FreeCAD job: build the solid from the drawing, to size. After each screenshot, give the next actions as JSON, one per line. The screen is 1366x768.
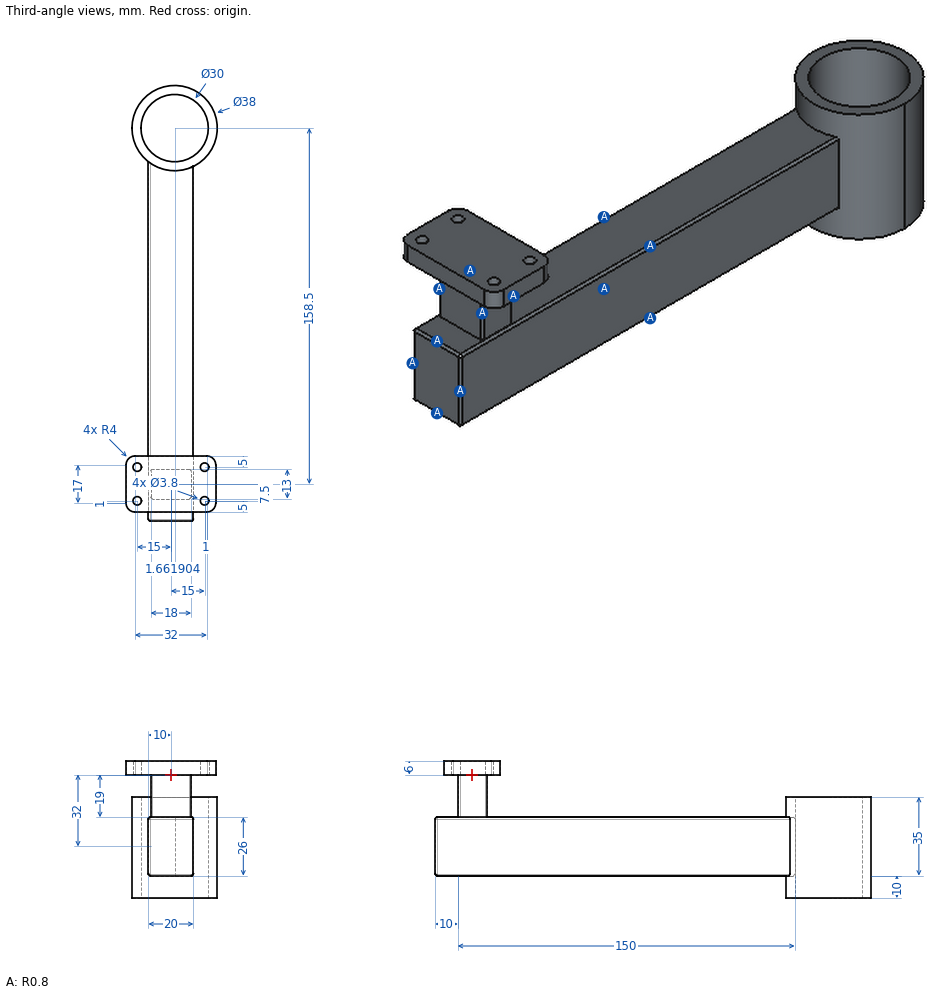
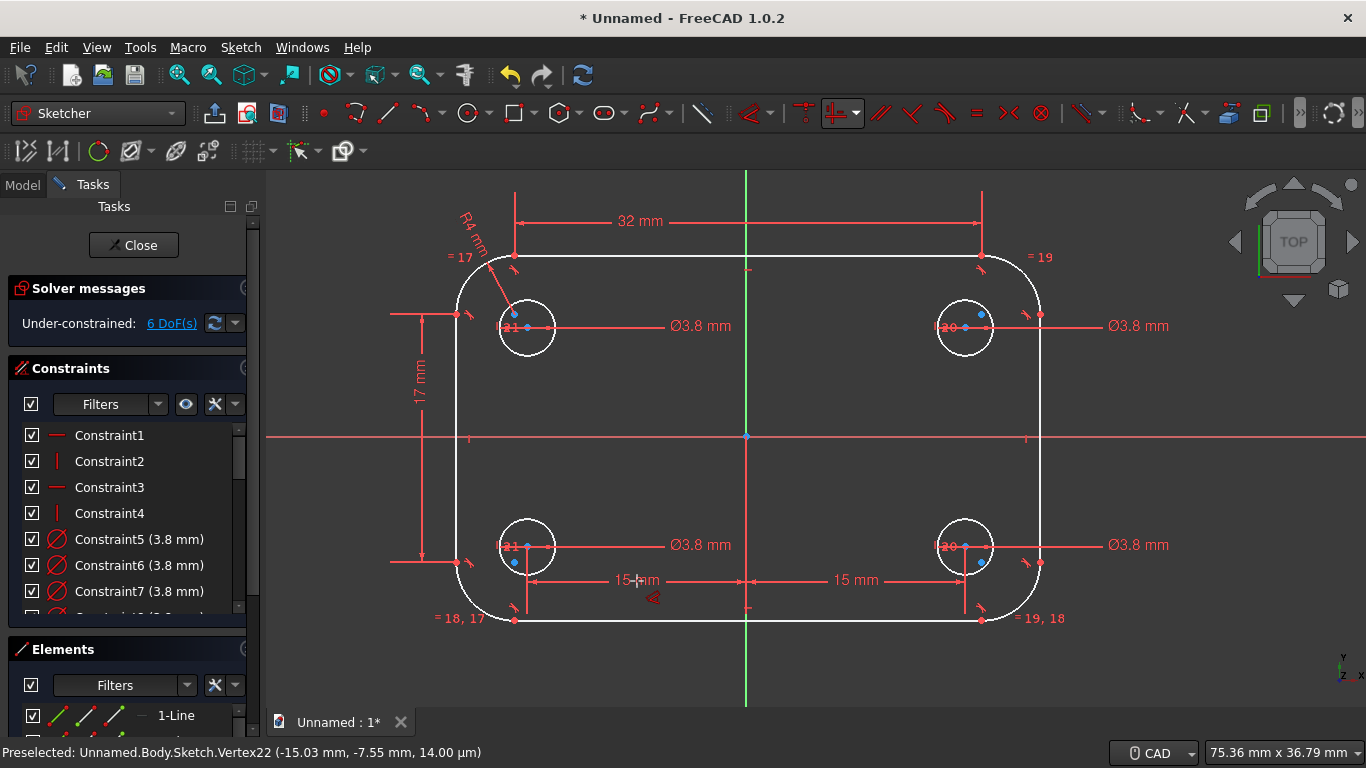
{"action": "scroll", "coordinate": [982, 621], "scroll_direction": "up", "scroll_amount": 6}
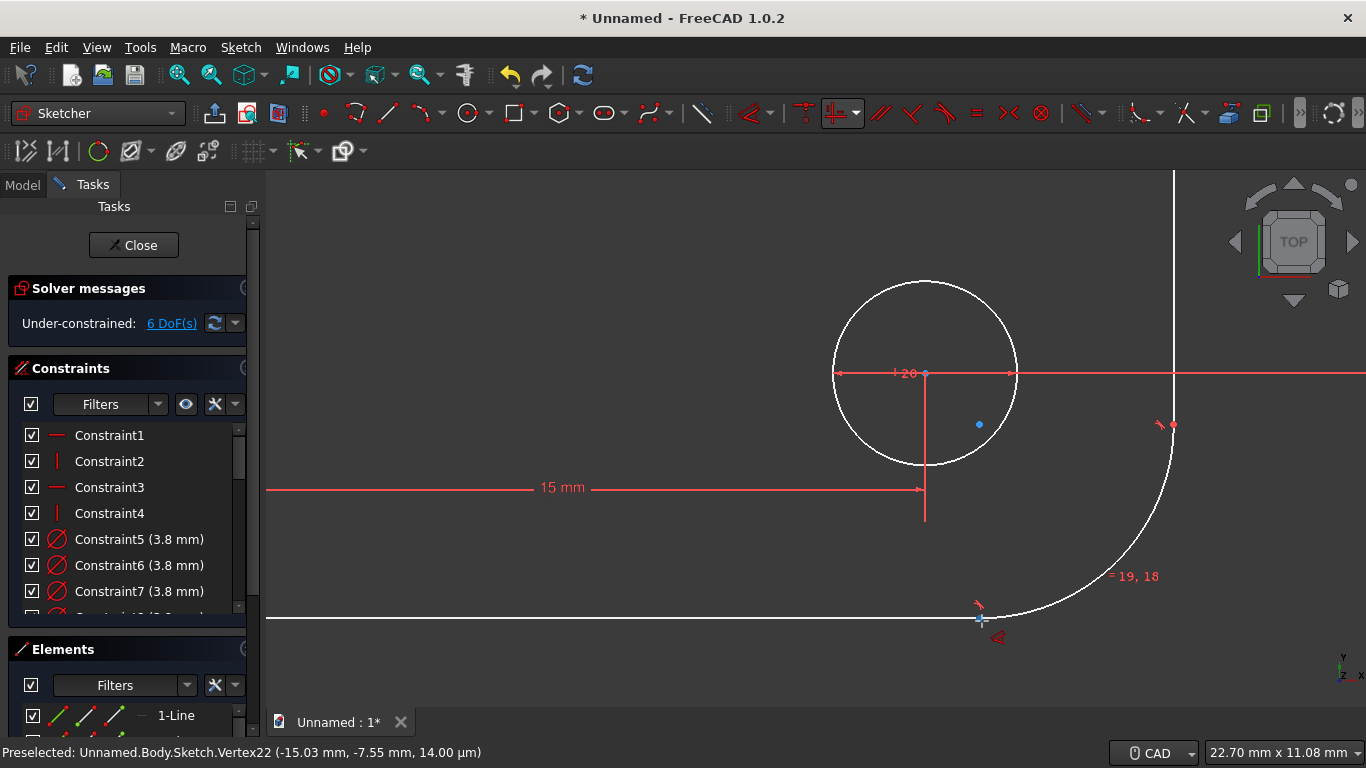
{"action": "left_click", "coordinate": [980, 618]}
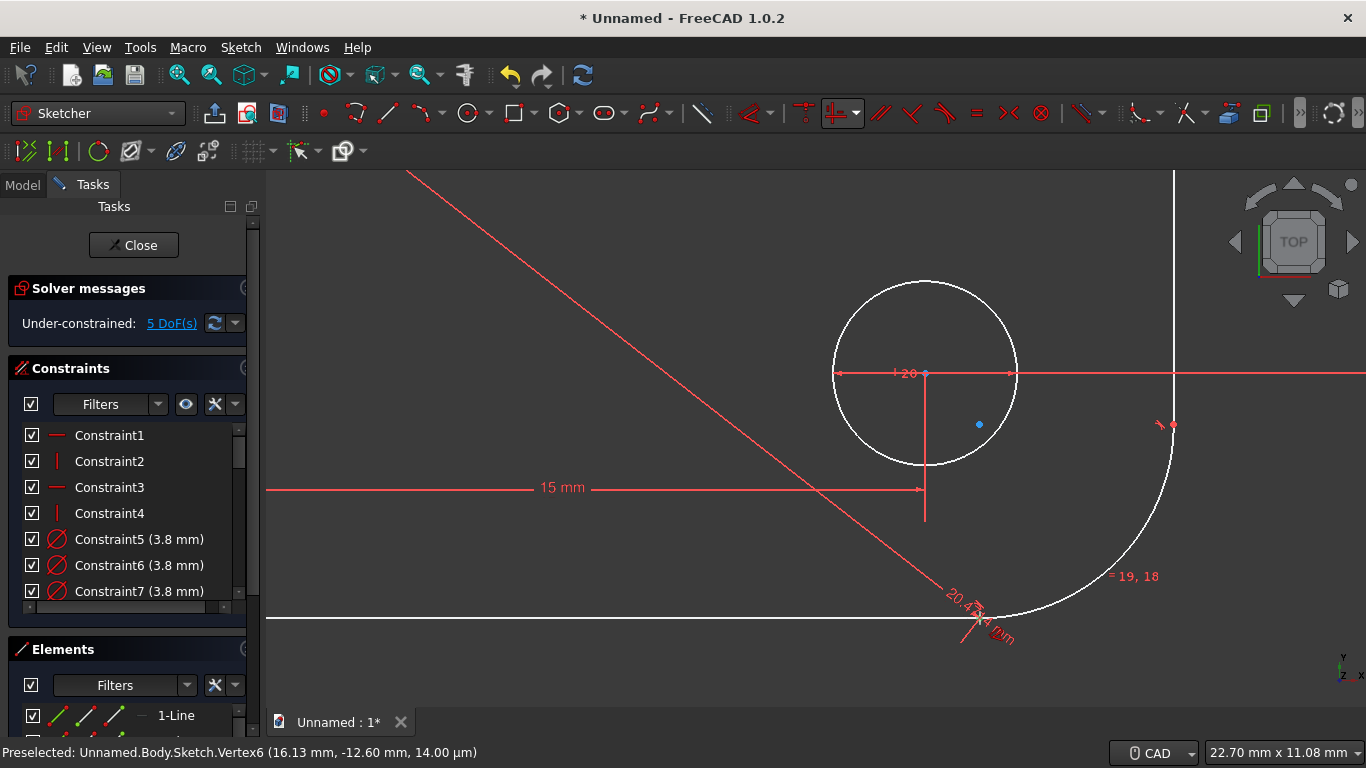
{"action": "left_click", "coordinate": [925, 373]}
{"action": "left_click", "coordinate": [952, 652]}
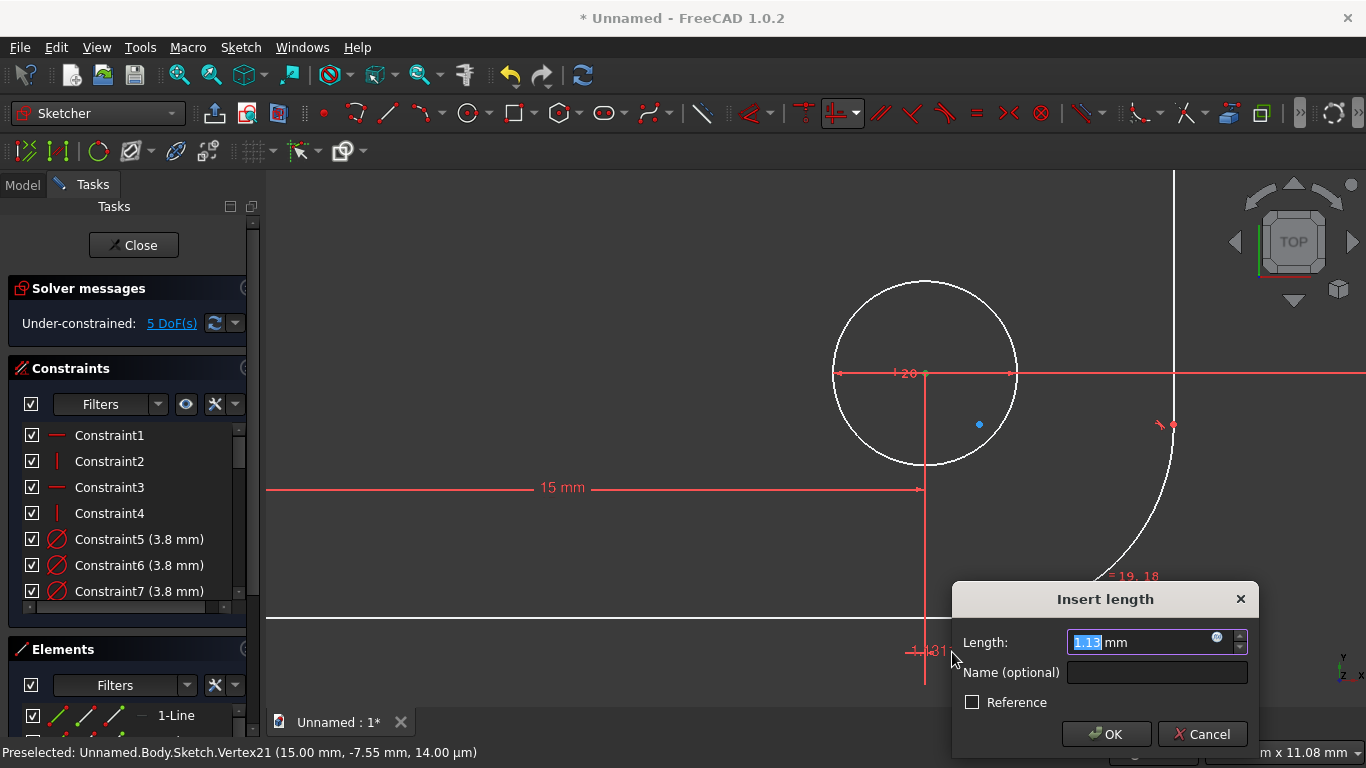
{"action": "type", "text": "1"}
{"action": "key", "text": "Return"}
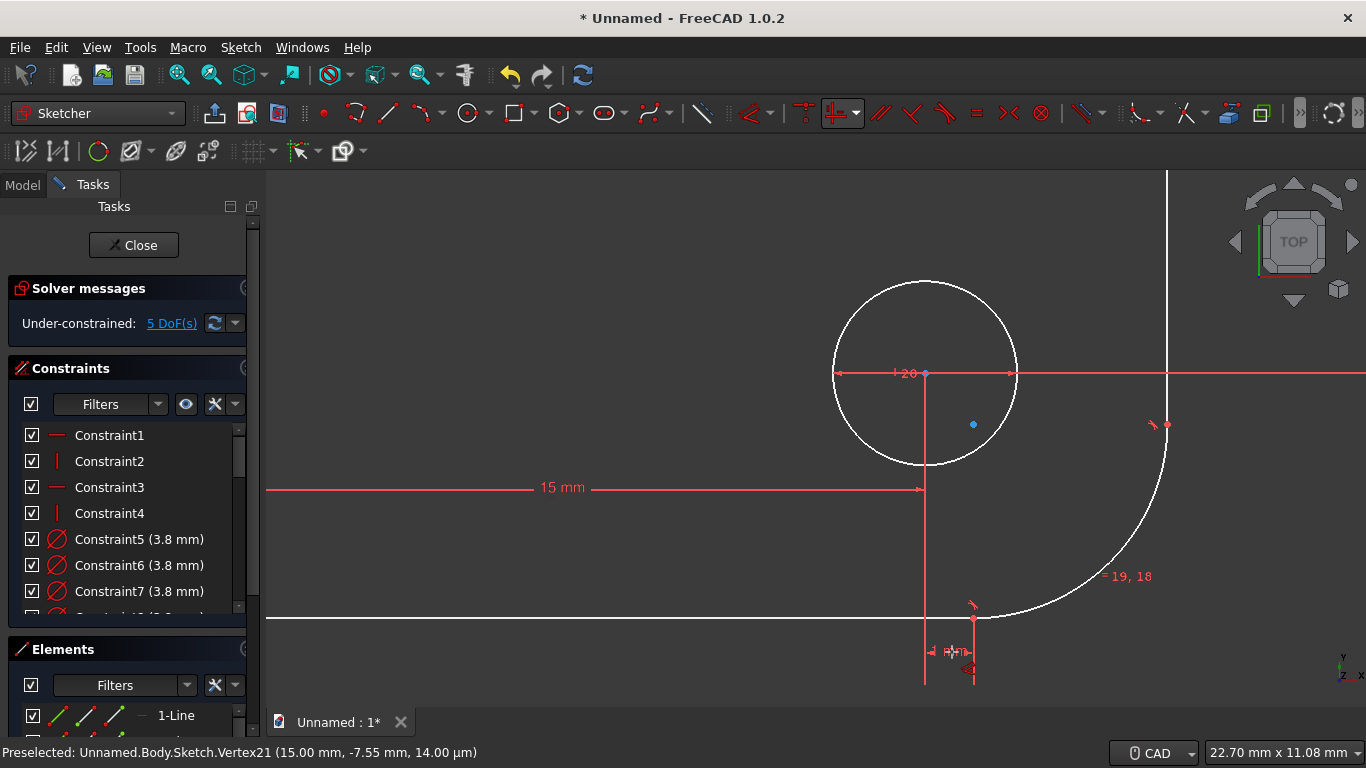
{"action": "left_click", "coordinate": [974, 618]}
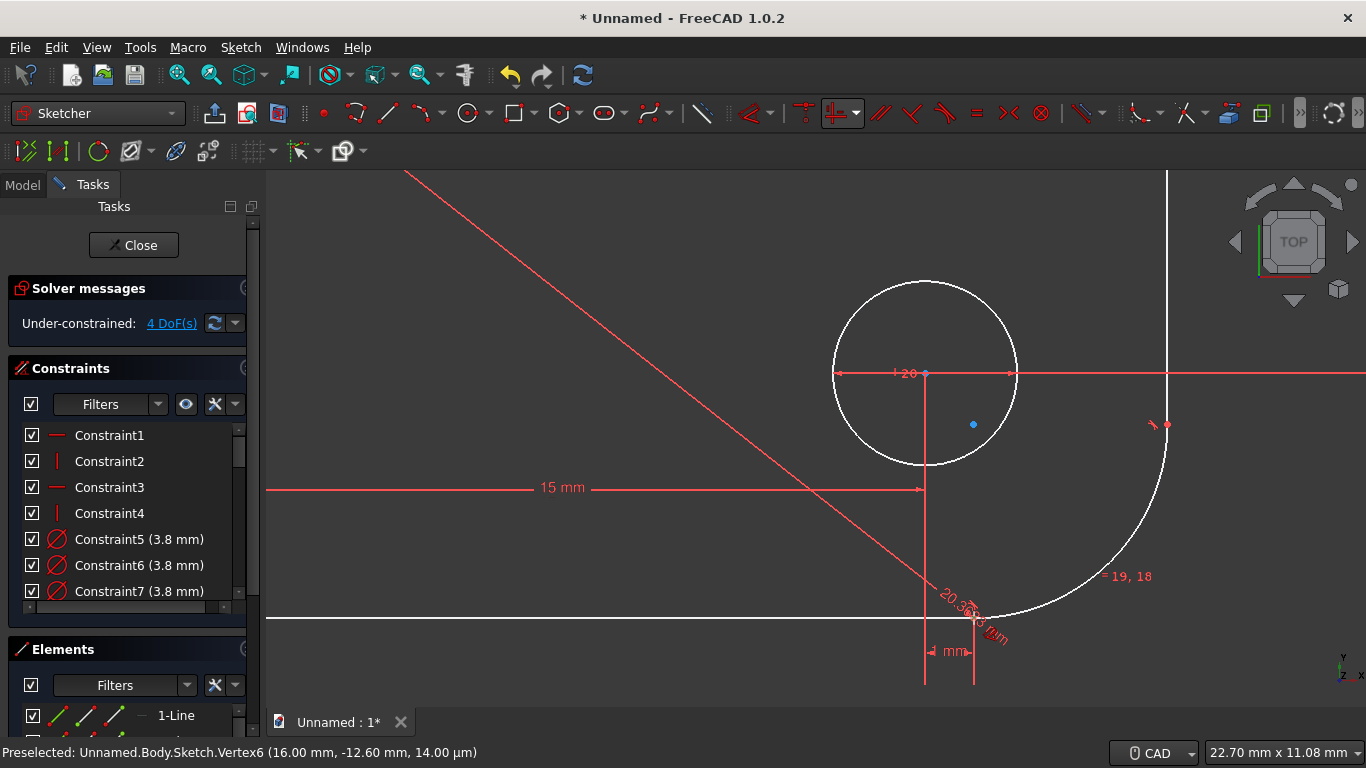
{"action": "left_click", "coordinate": [925, 373]}
{"action": "left_click", "coordinate": [1008, 496]}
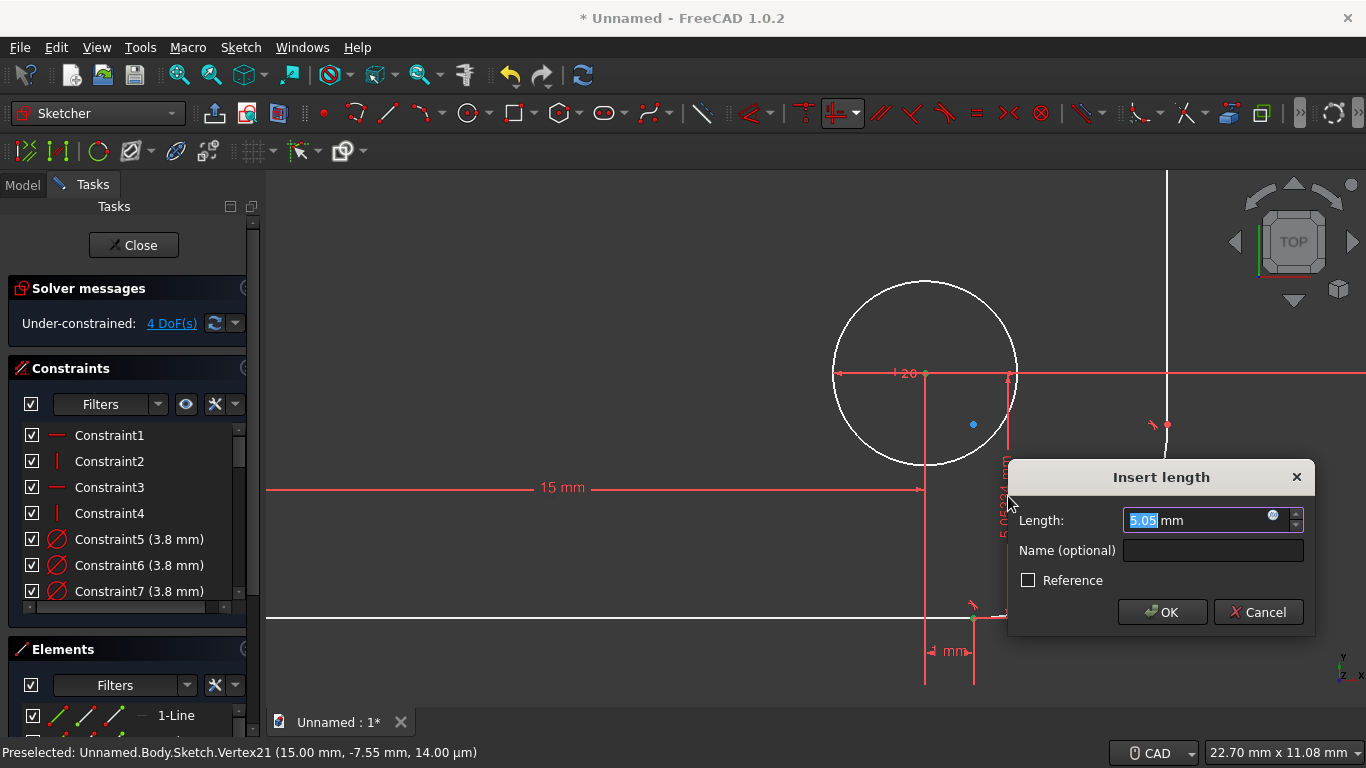
{"action": "type", "text": "5"}
{"action": "key", "text": "Return"}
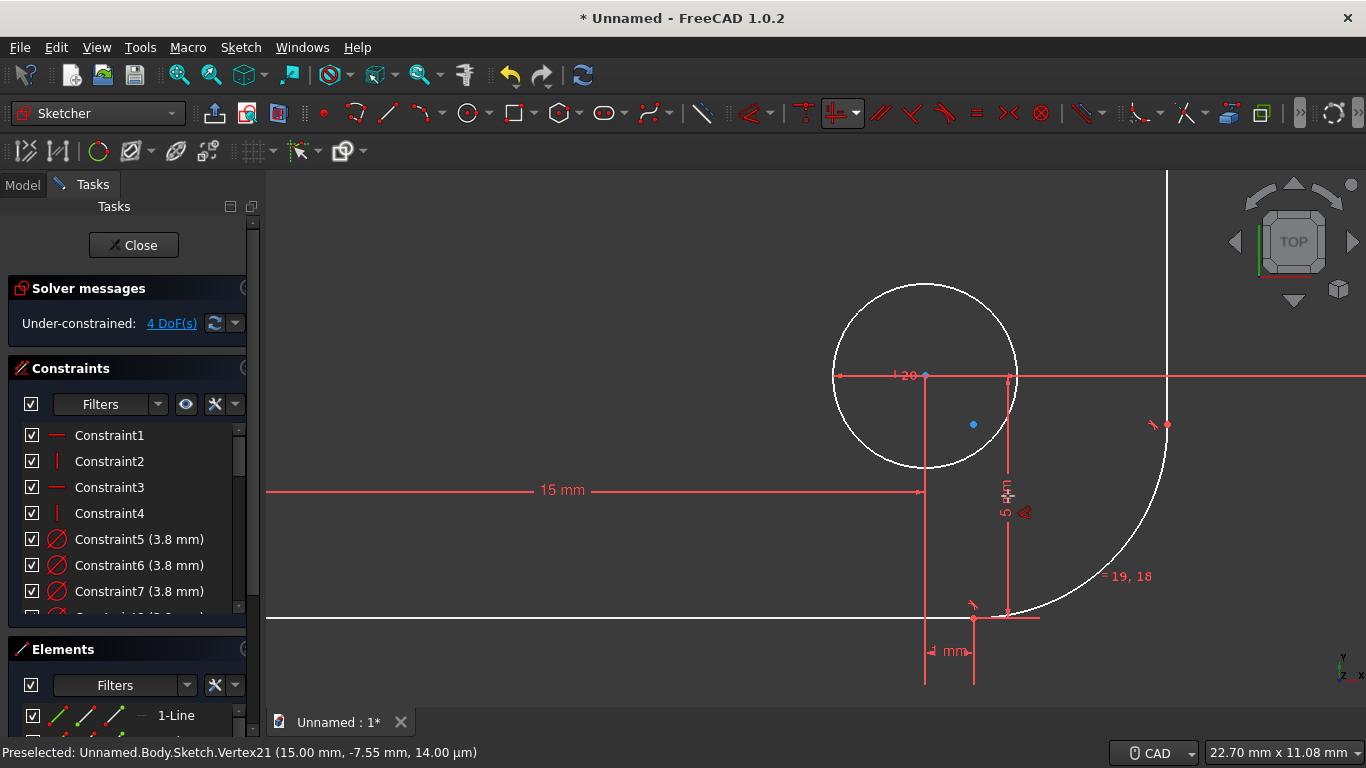
{"action": "scroll", "coordinate": [984, 624], "scroll_direction": "down", "scroll_amount": 6}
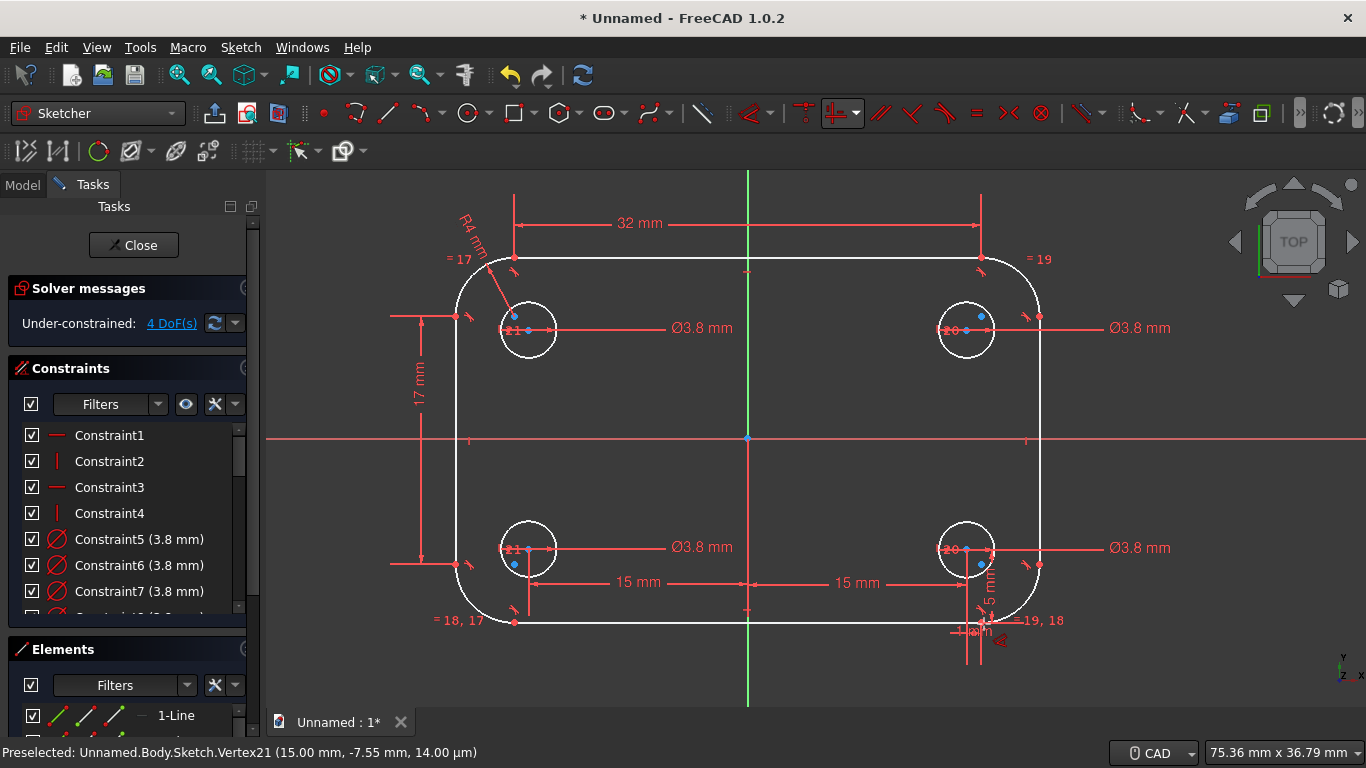
{"action": "scroll", "coordinate": [456, 564], "scroll_direction": "up", "scroll_amount": 6}